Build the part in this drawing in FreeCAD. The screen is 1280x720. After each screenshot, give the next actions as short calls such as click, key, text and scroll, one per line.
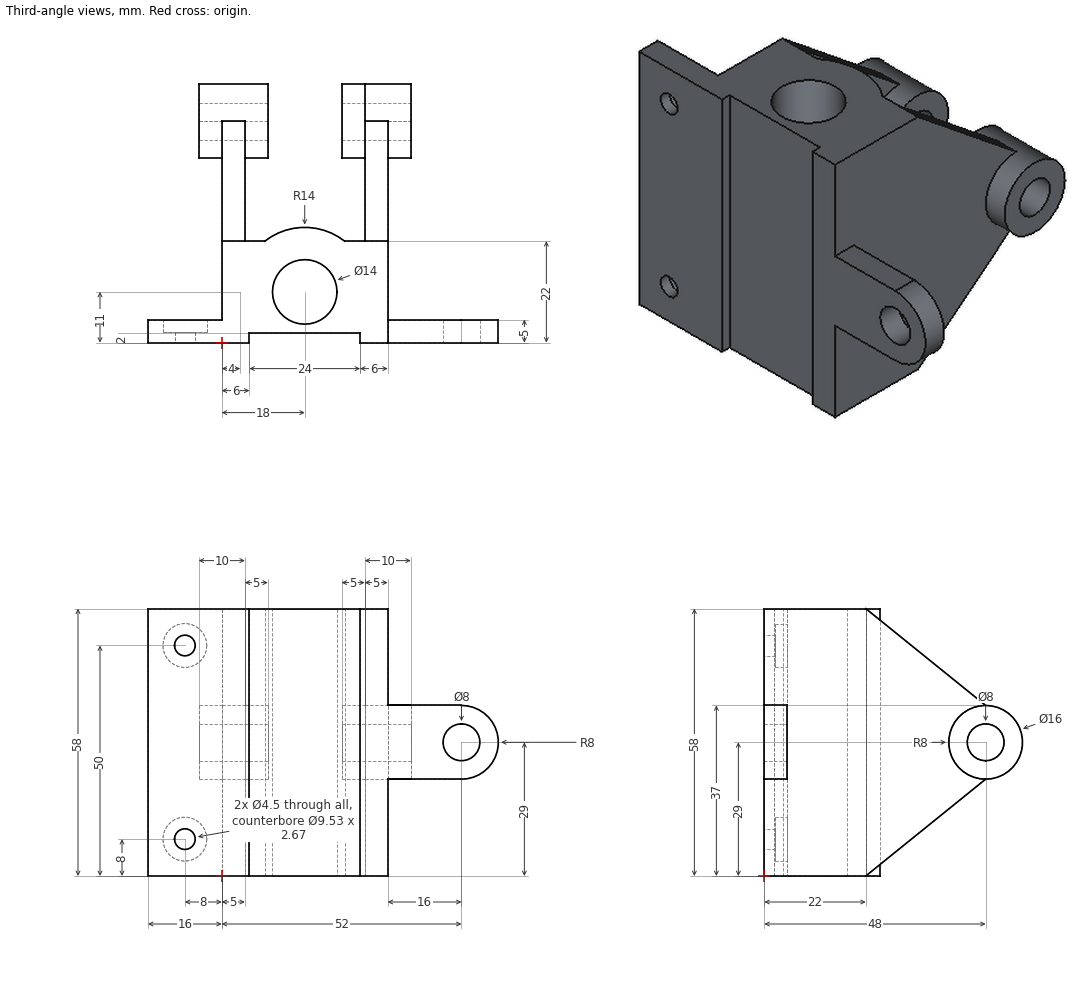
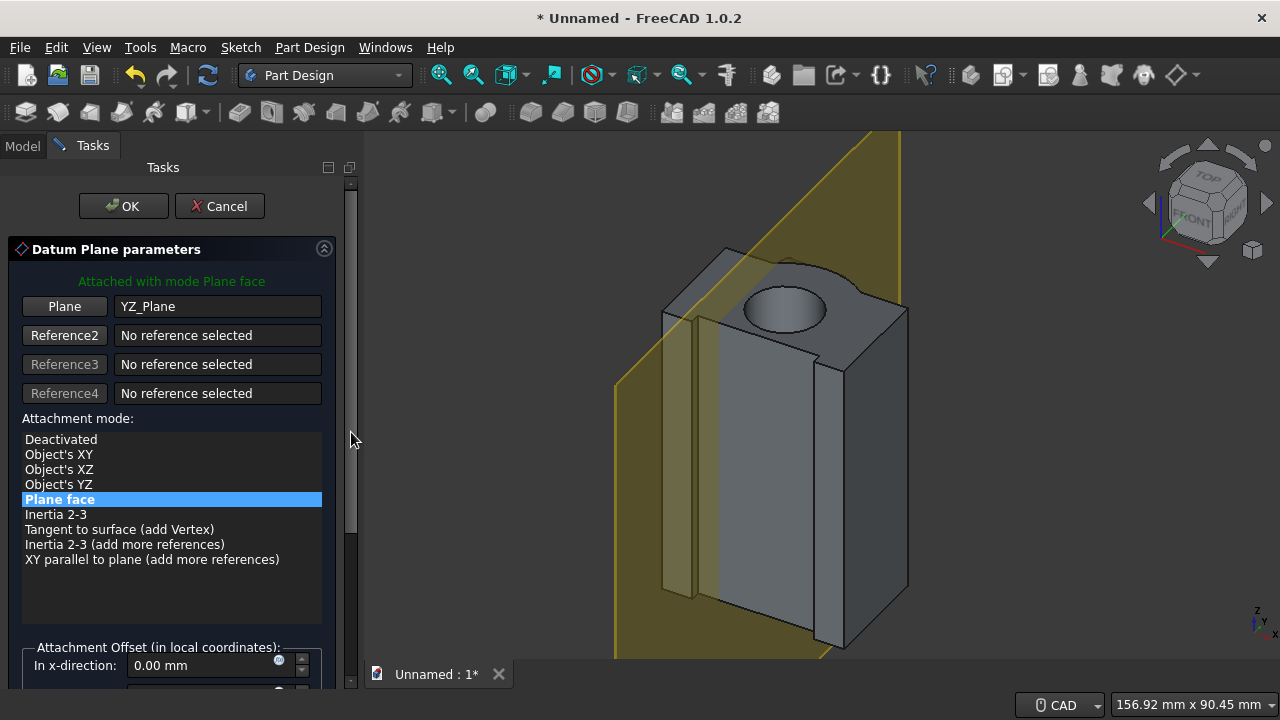
click(124, 206)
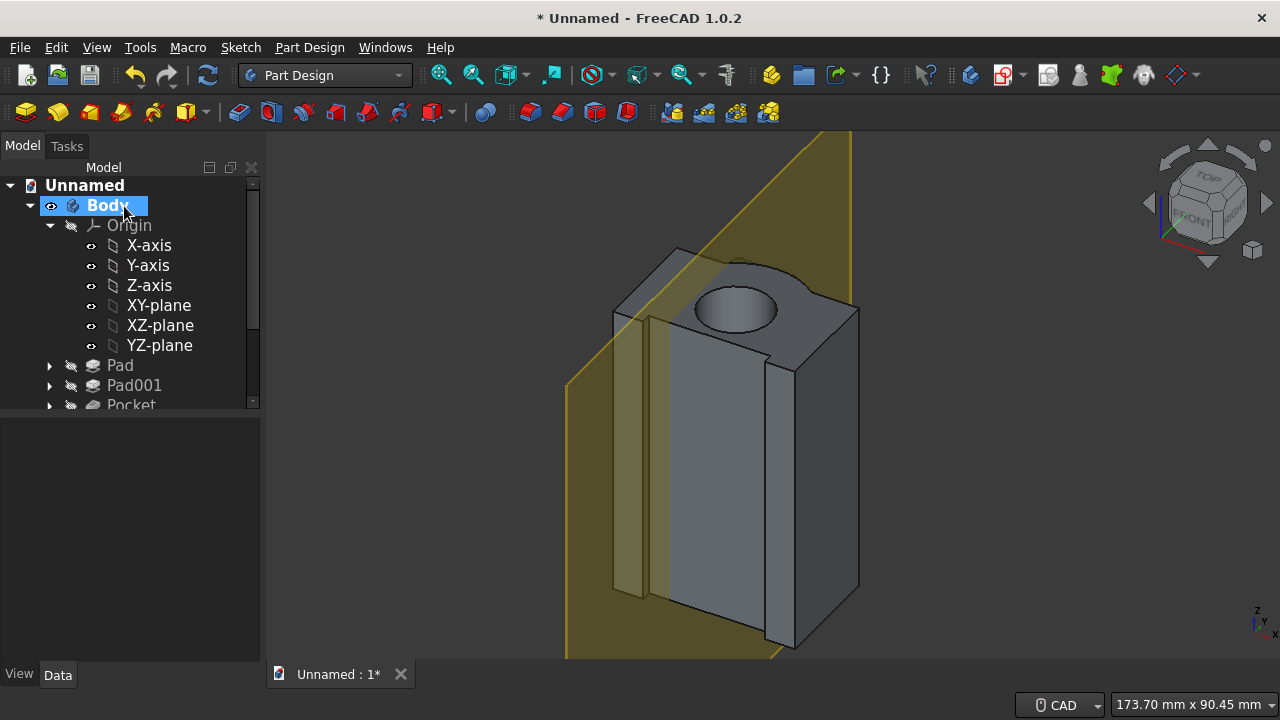
scroll(100, 301, down, 3)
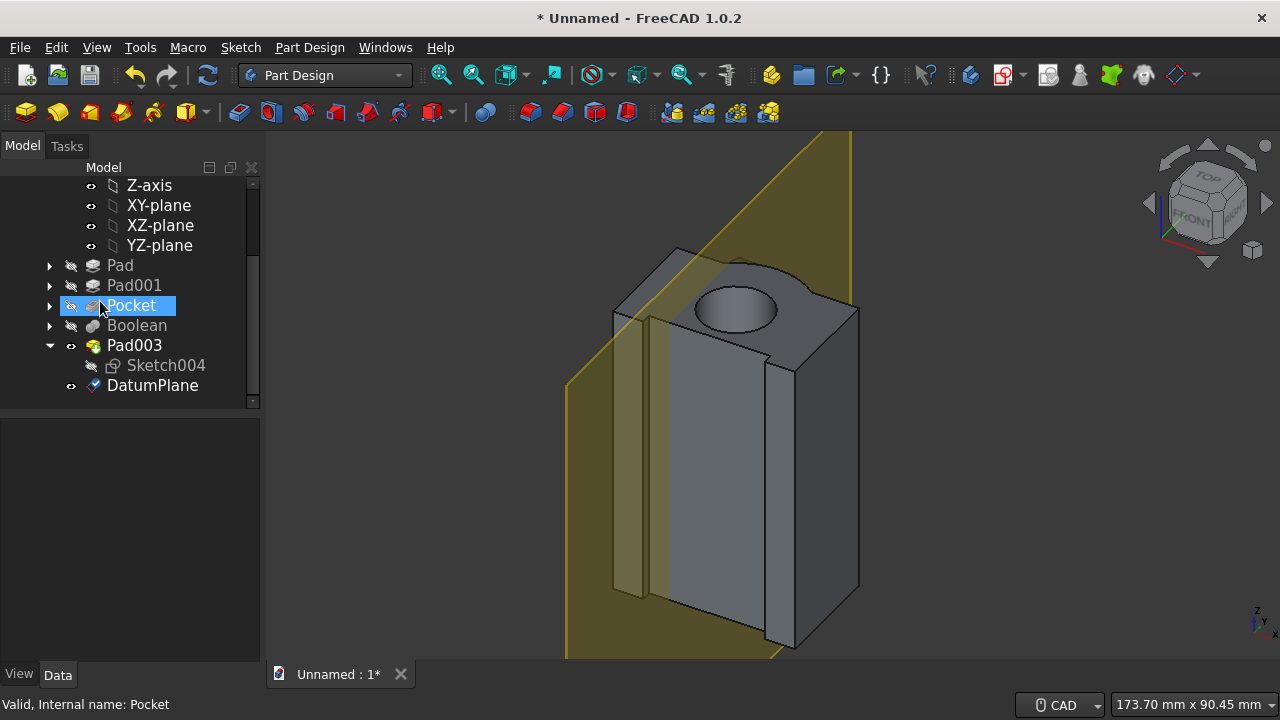
click(116, 386)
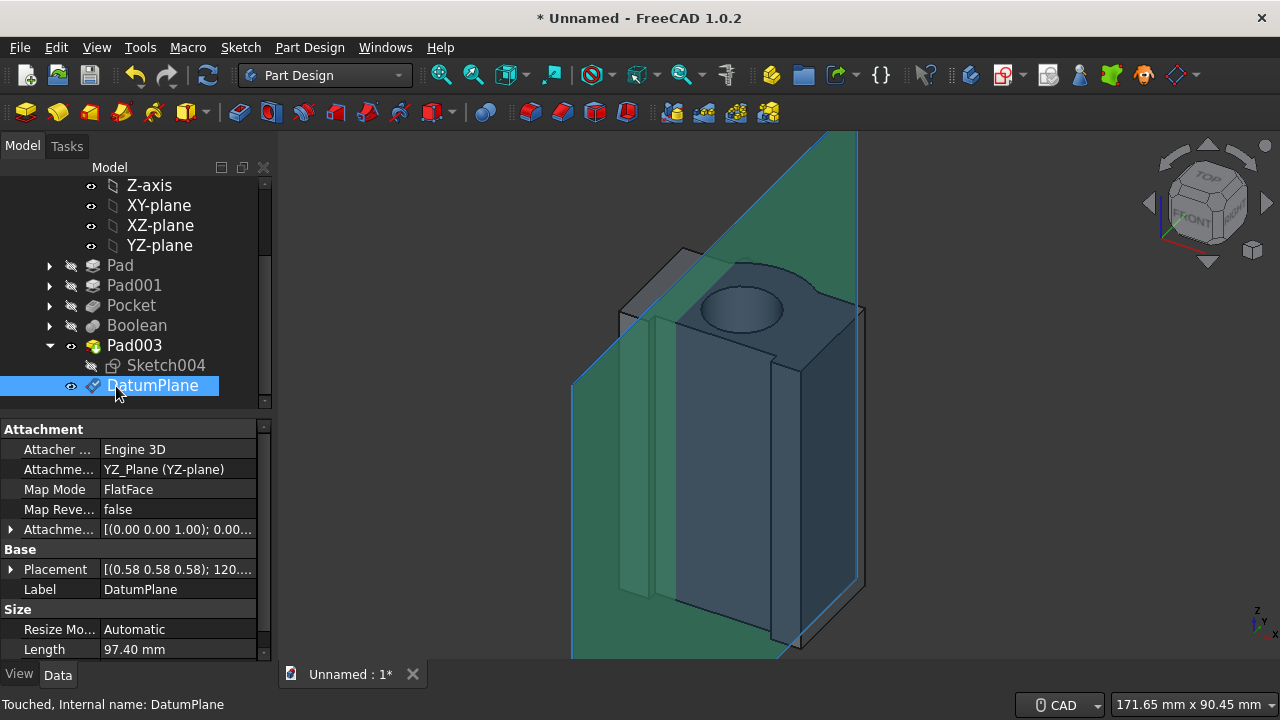
click(1004, 76)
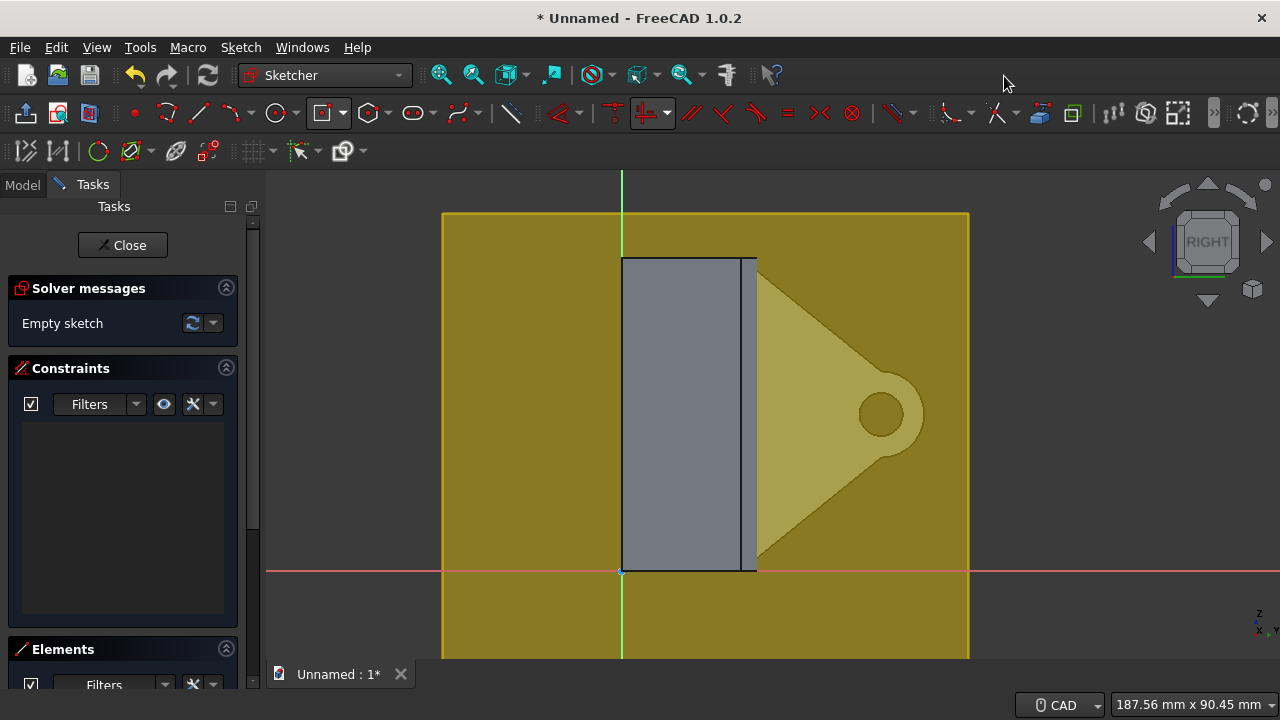
key(q)
key(s)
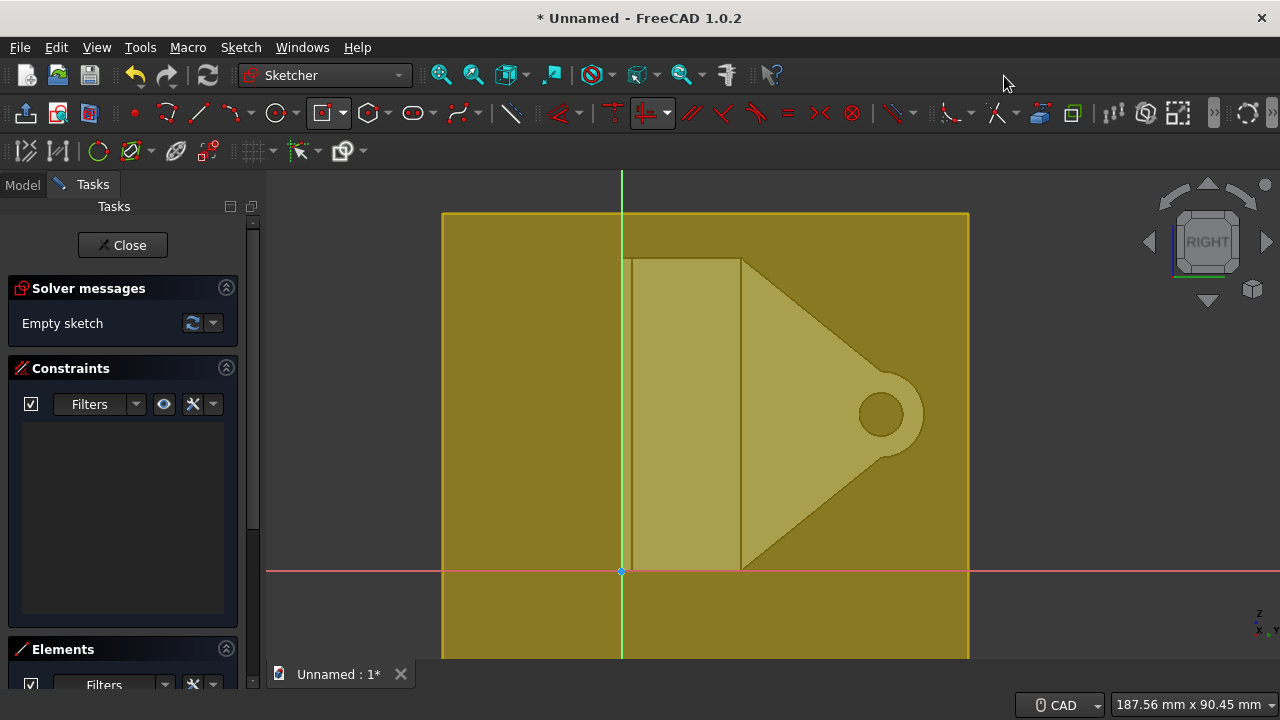
scroll(957, 415, up, 6)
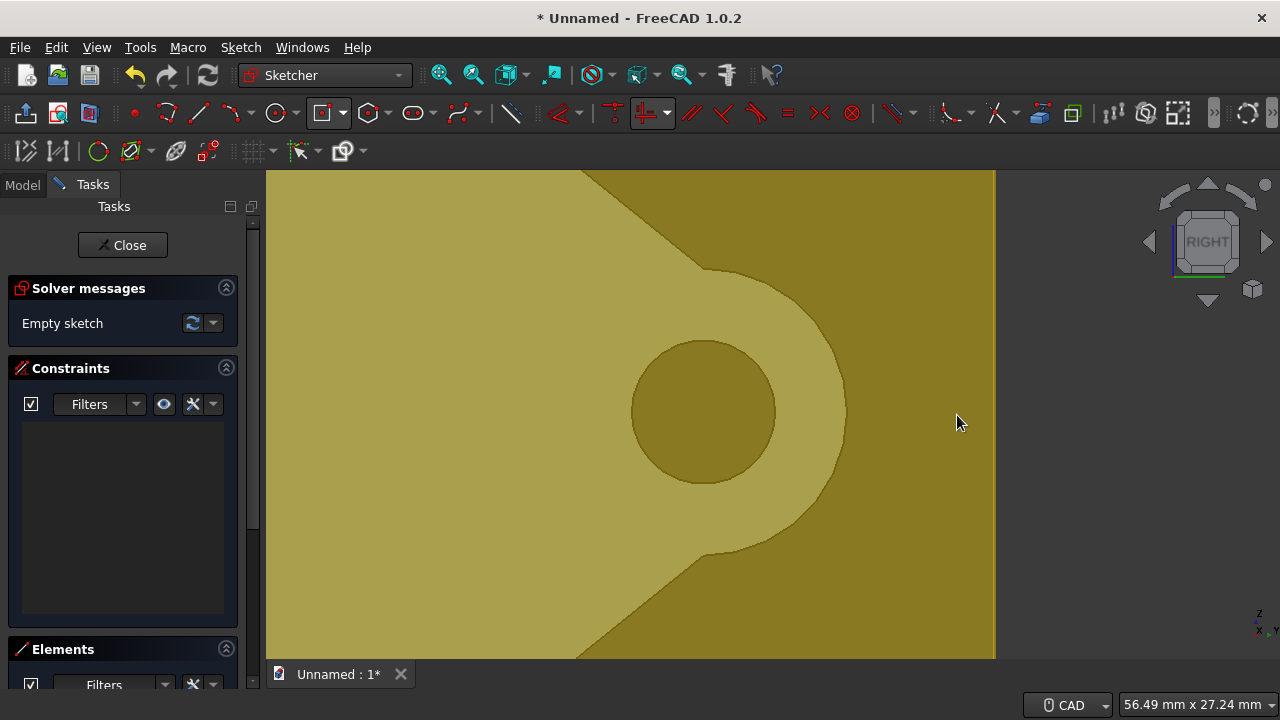
key(g)
key(c)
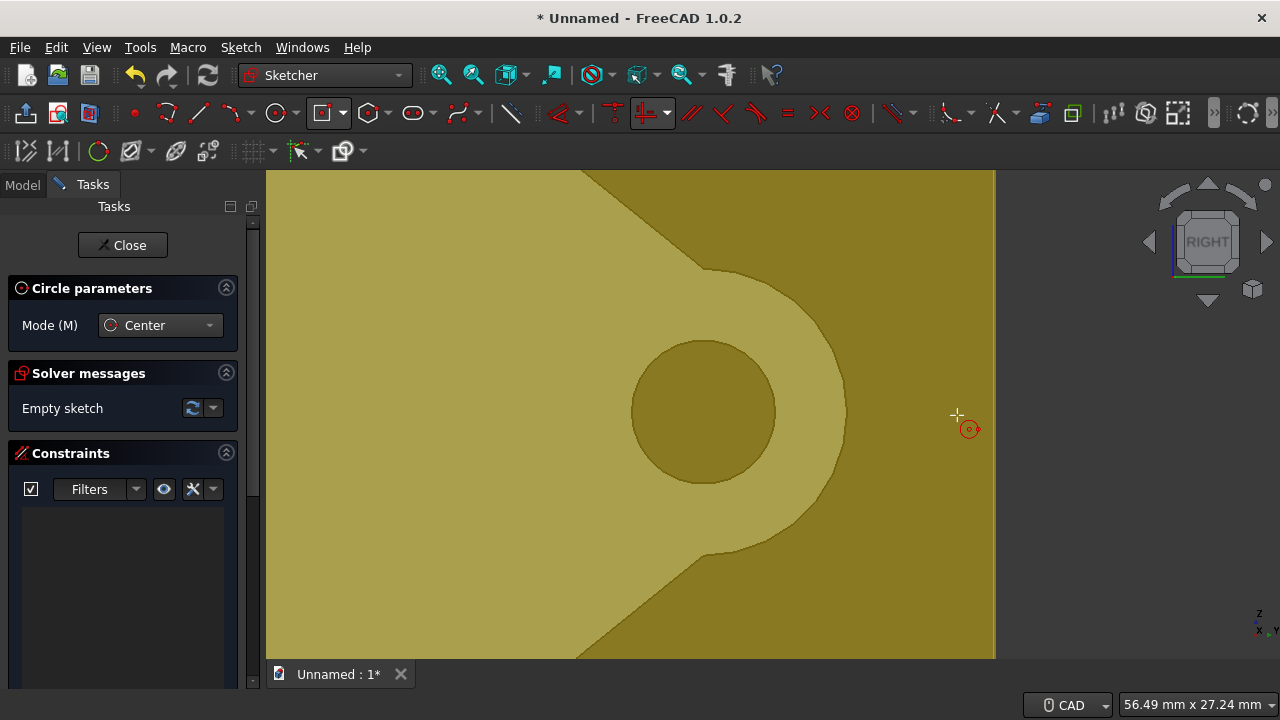
click(704, 412)
move(805, 311)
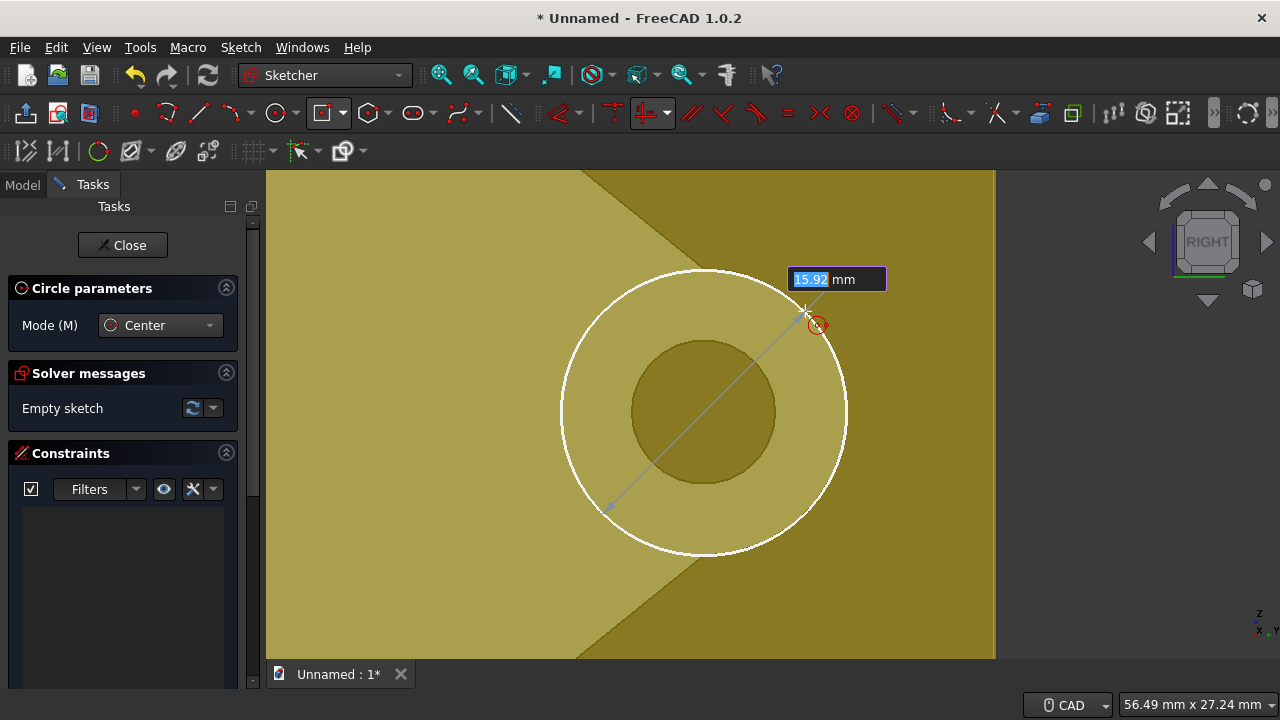
text(16)
key(Return)
key(Escape)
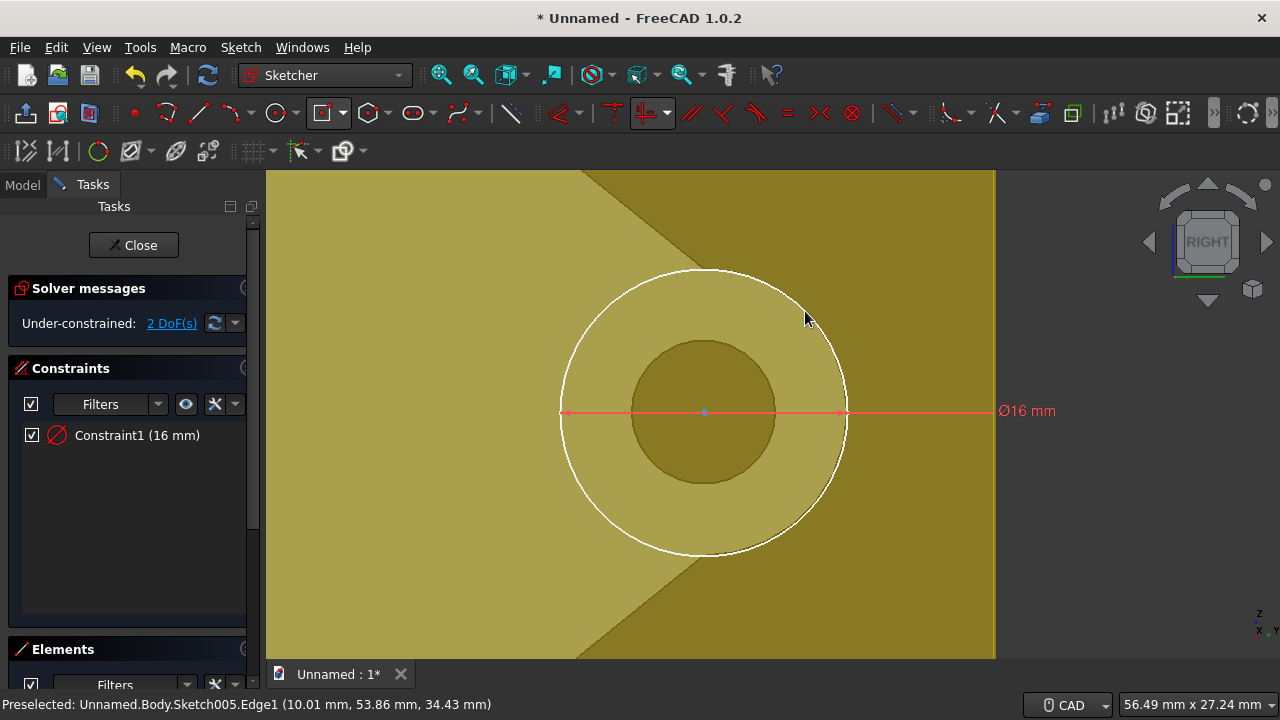
key(d)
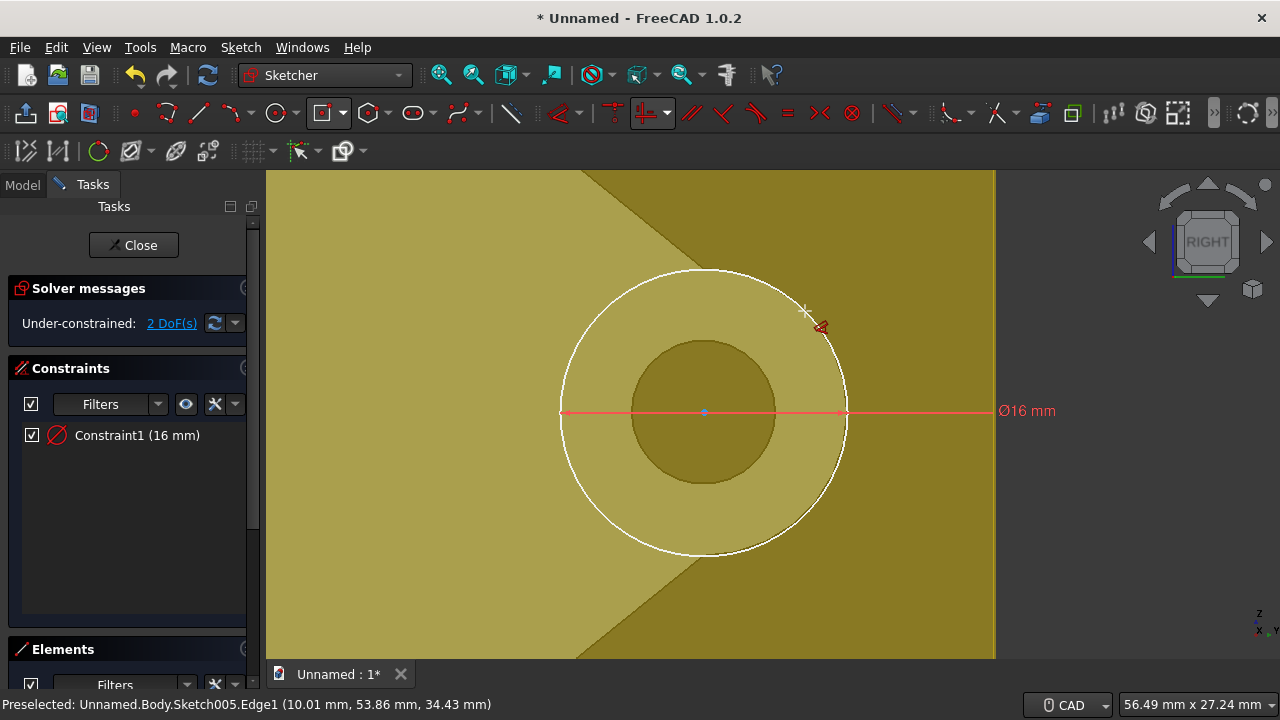
click(704, 413)
click(499, 379)